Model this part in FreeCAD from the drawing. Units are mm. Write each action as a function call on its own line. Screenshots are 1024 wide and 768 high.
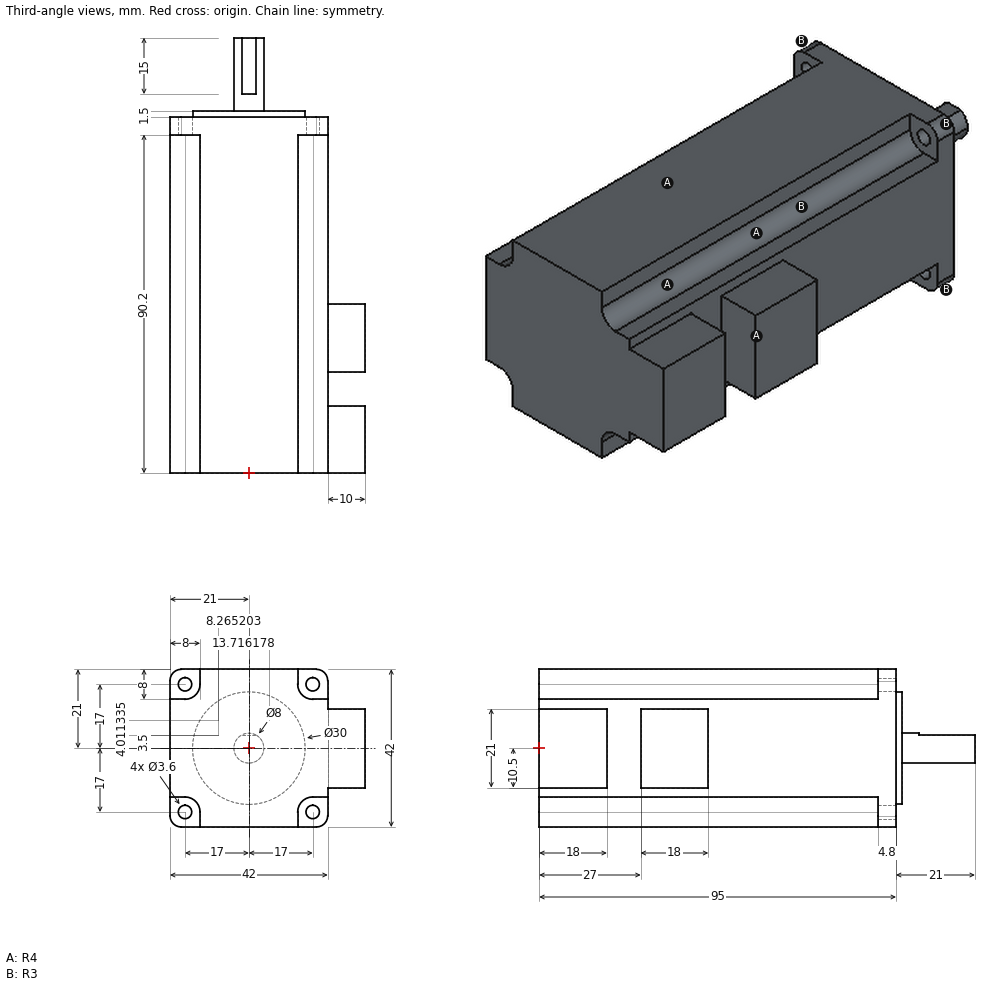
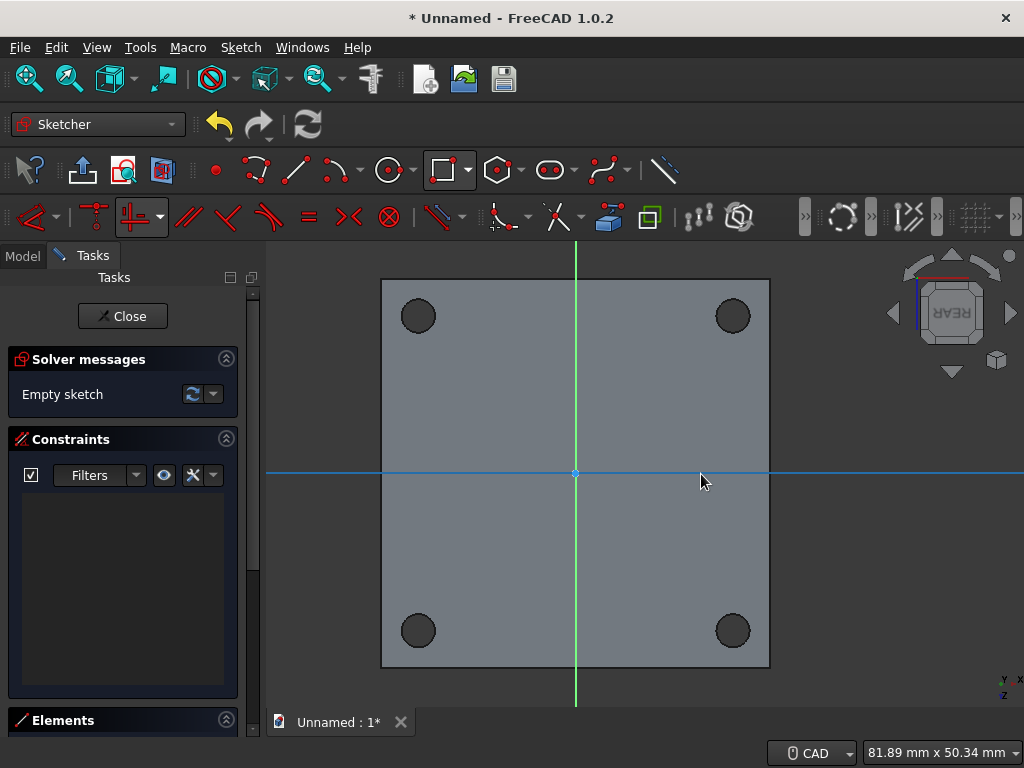
key(g)
key(c)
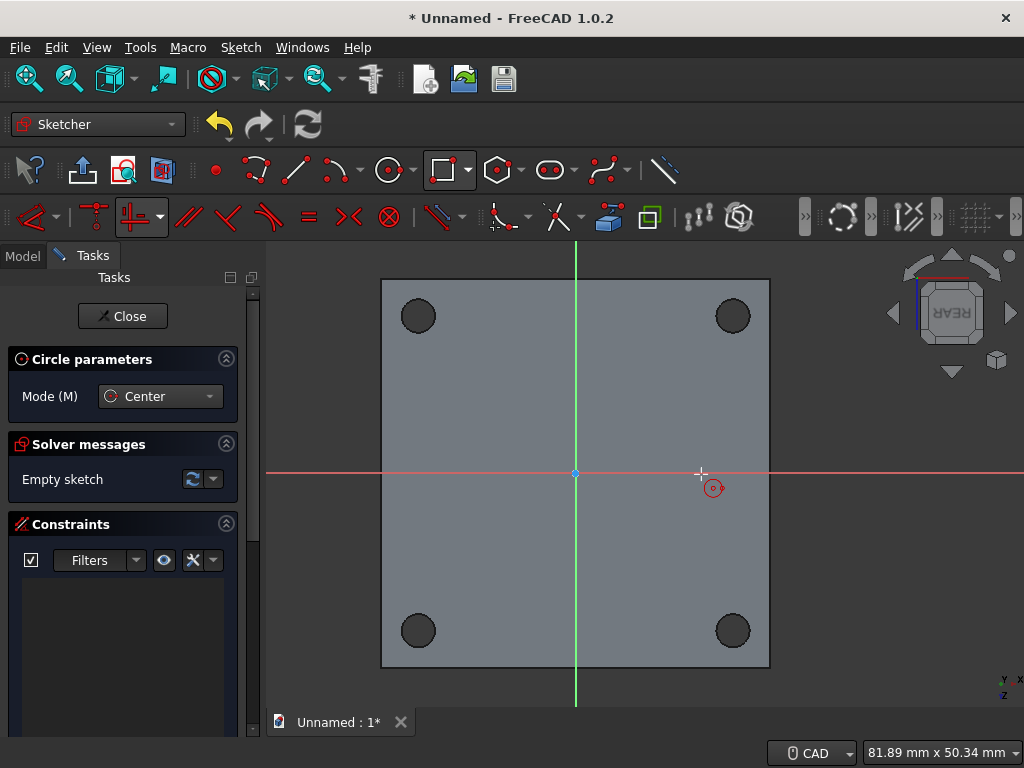
click(576, 473)
click(674, 375)
key(Escape)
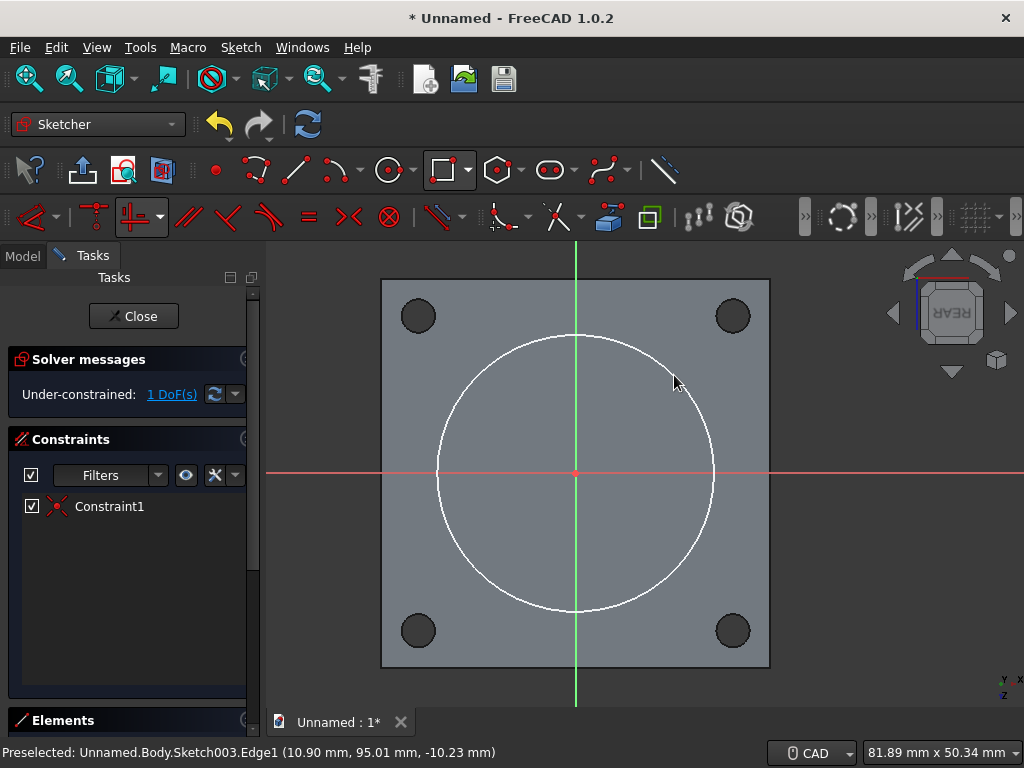
click(32, 218)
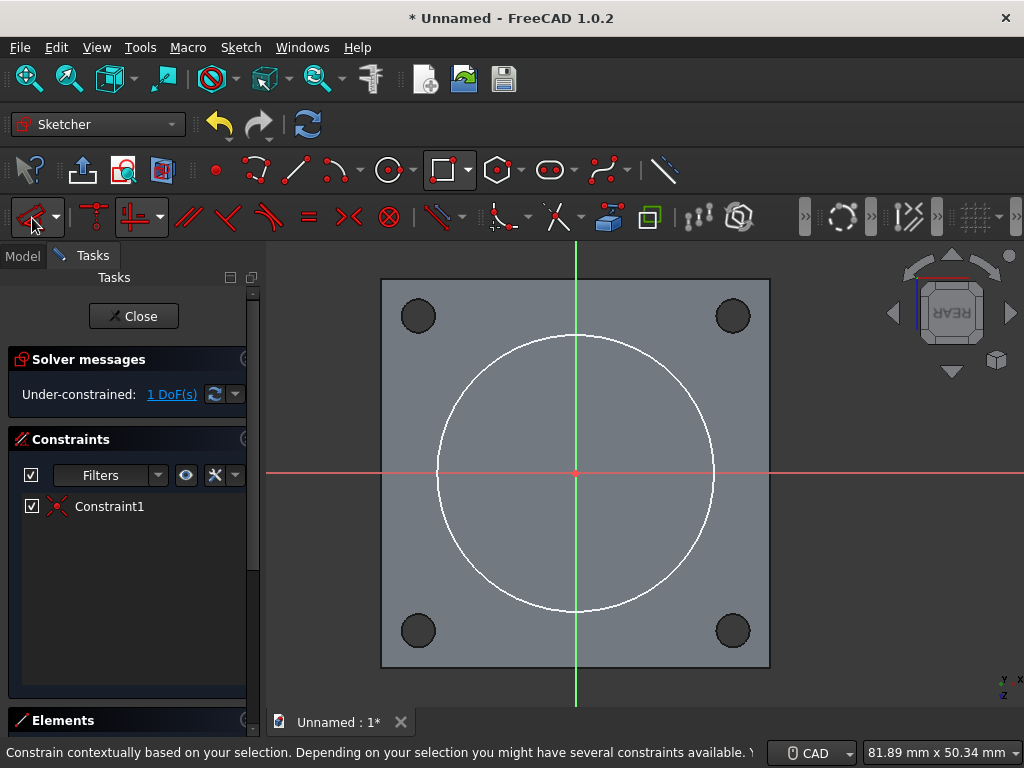
click(673, 375)
click(696, 352)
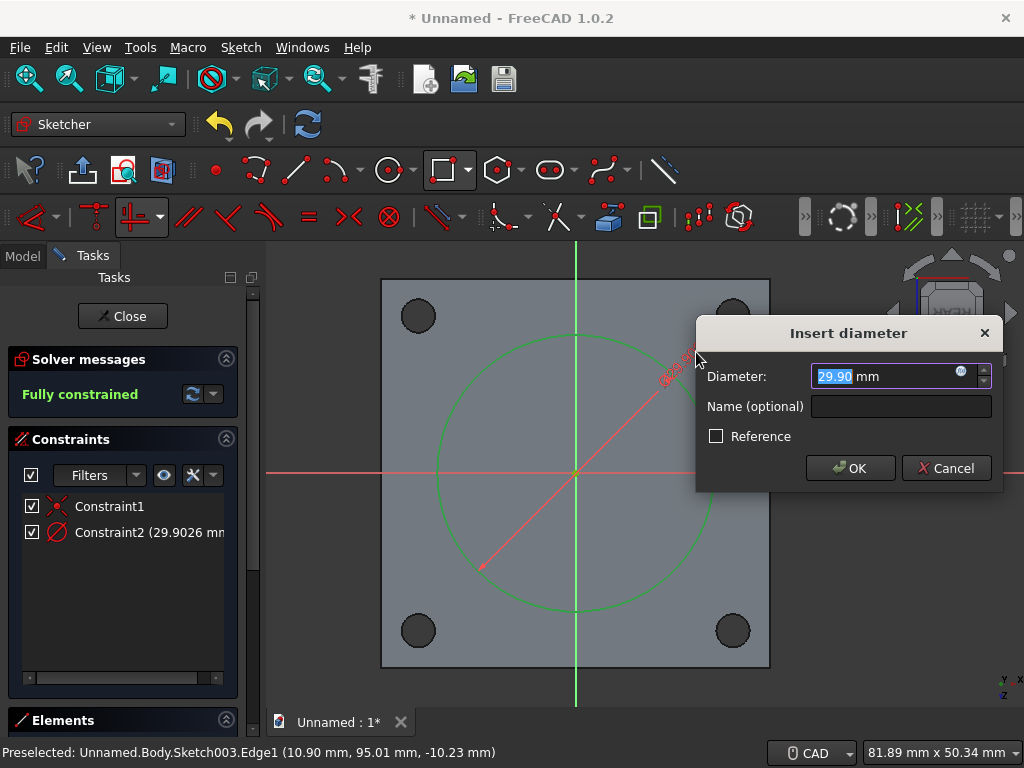
text(30)
key(Return)
key(Escape)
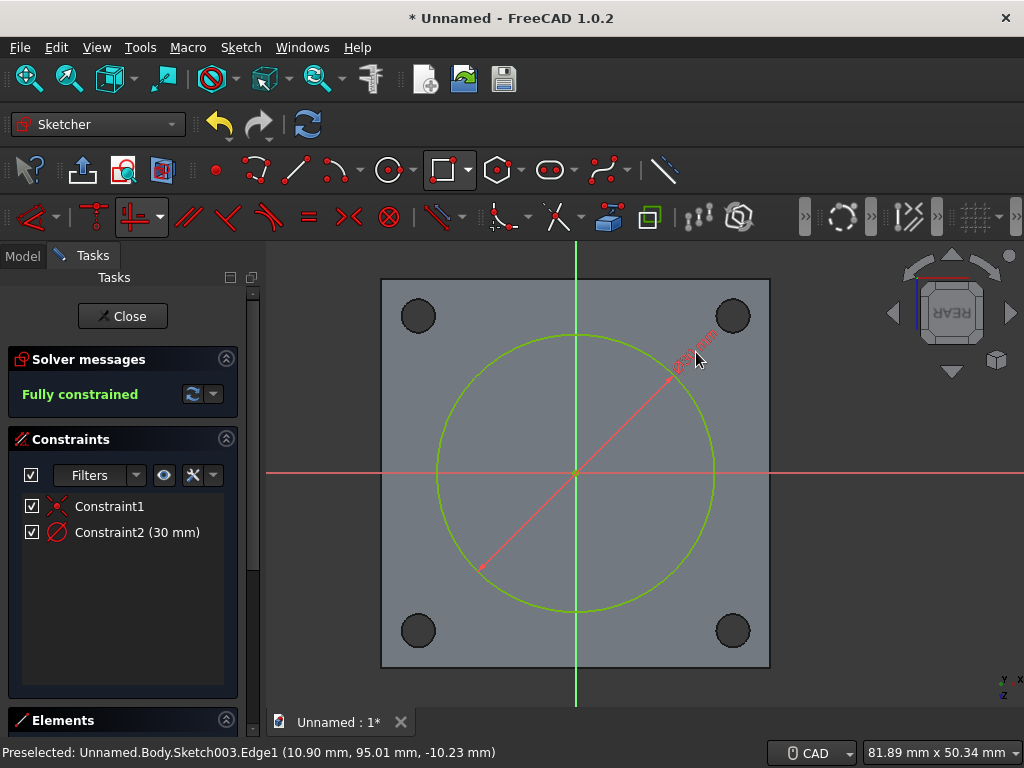
click(123, 316)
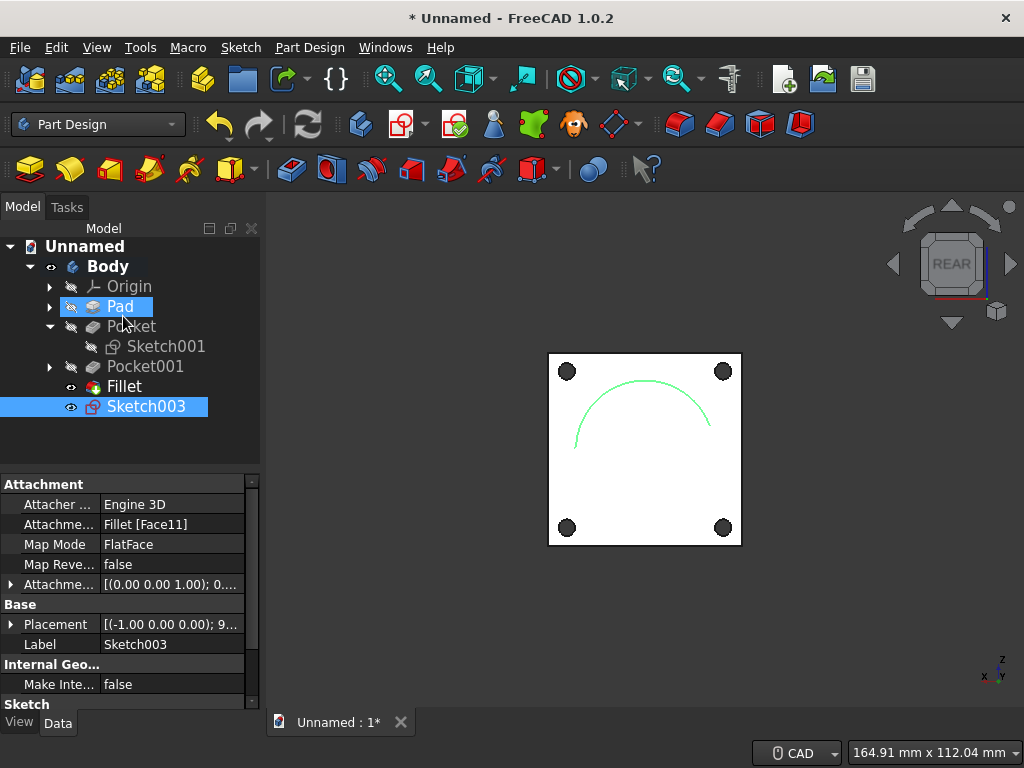
click(30, 170)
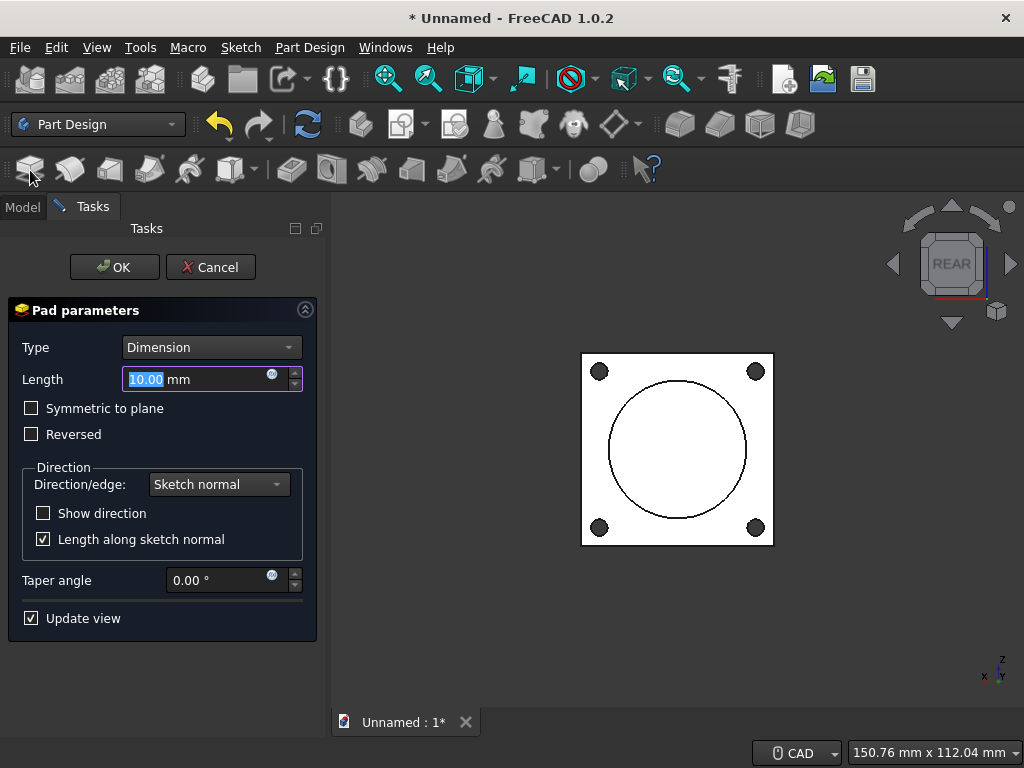
text(1.5)
key(Tab)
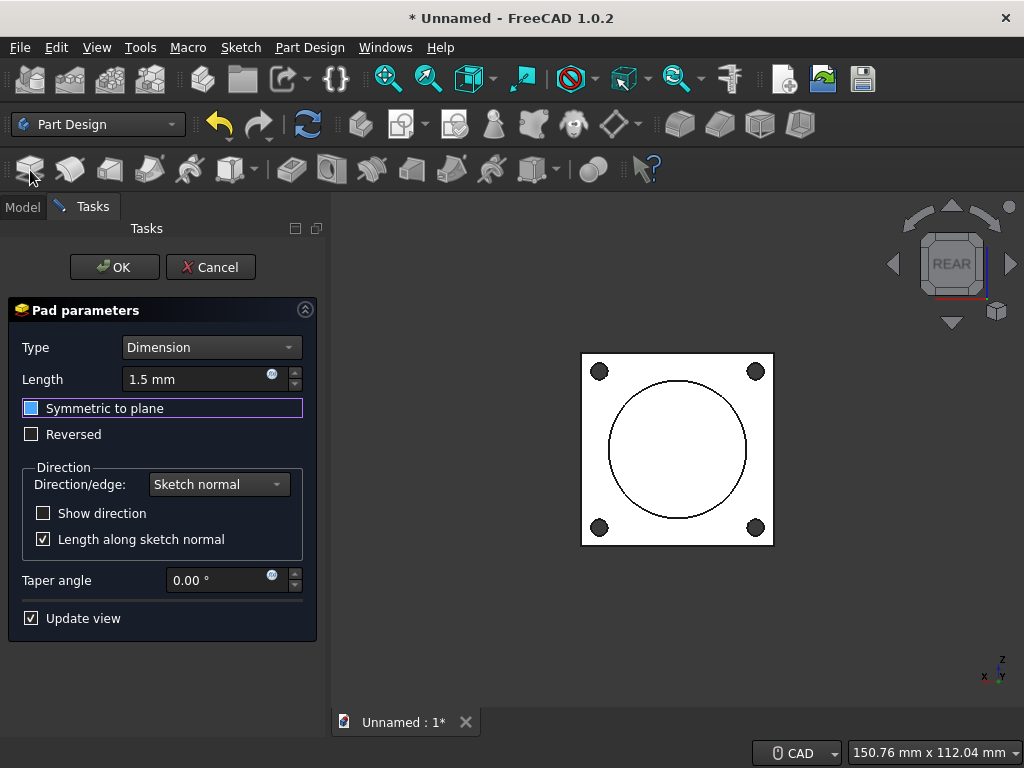
click(115, 267)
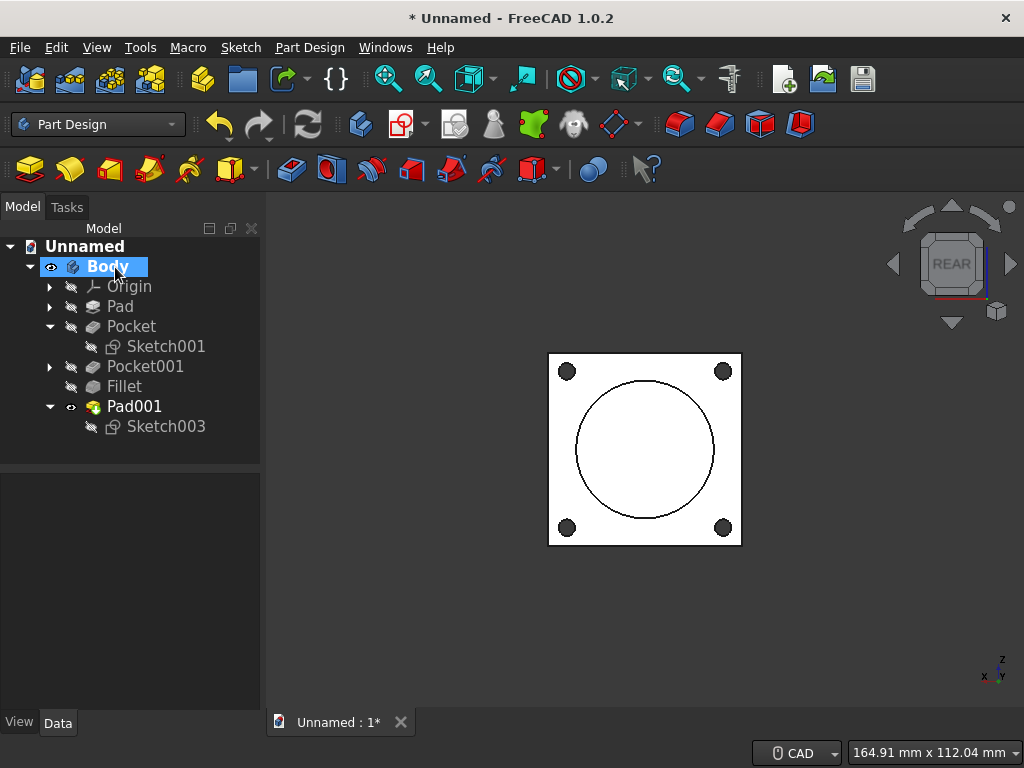
key(v)
key(f)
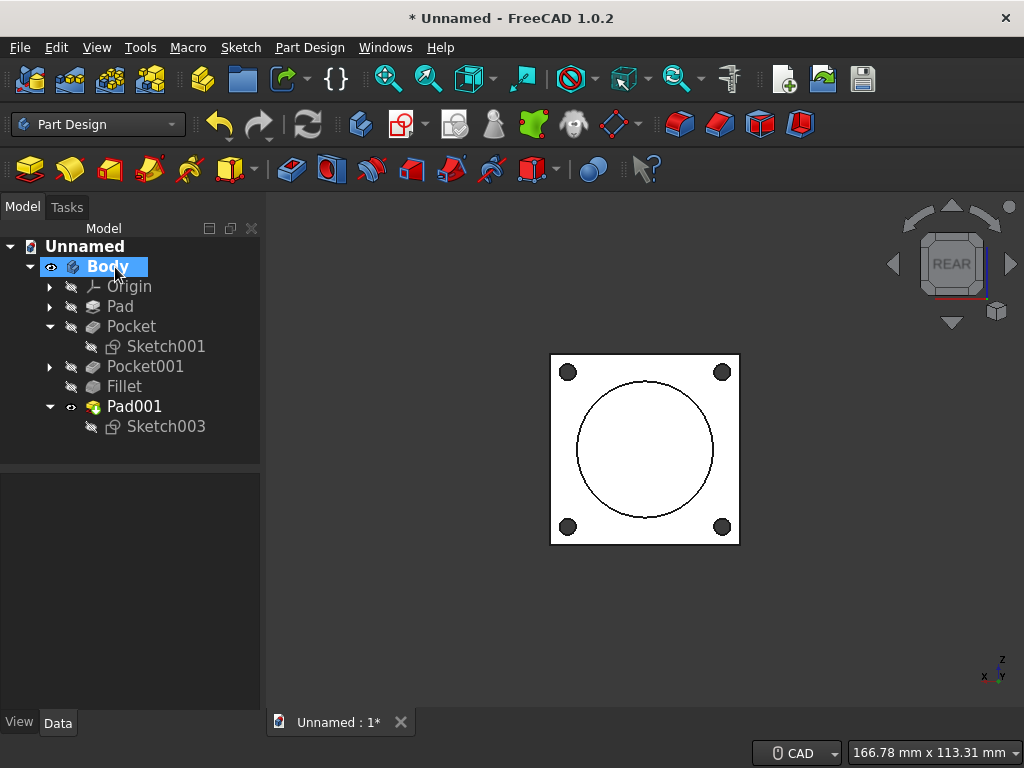
click(563, 394)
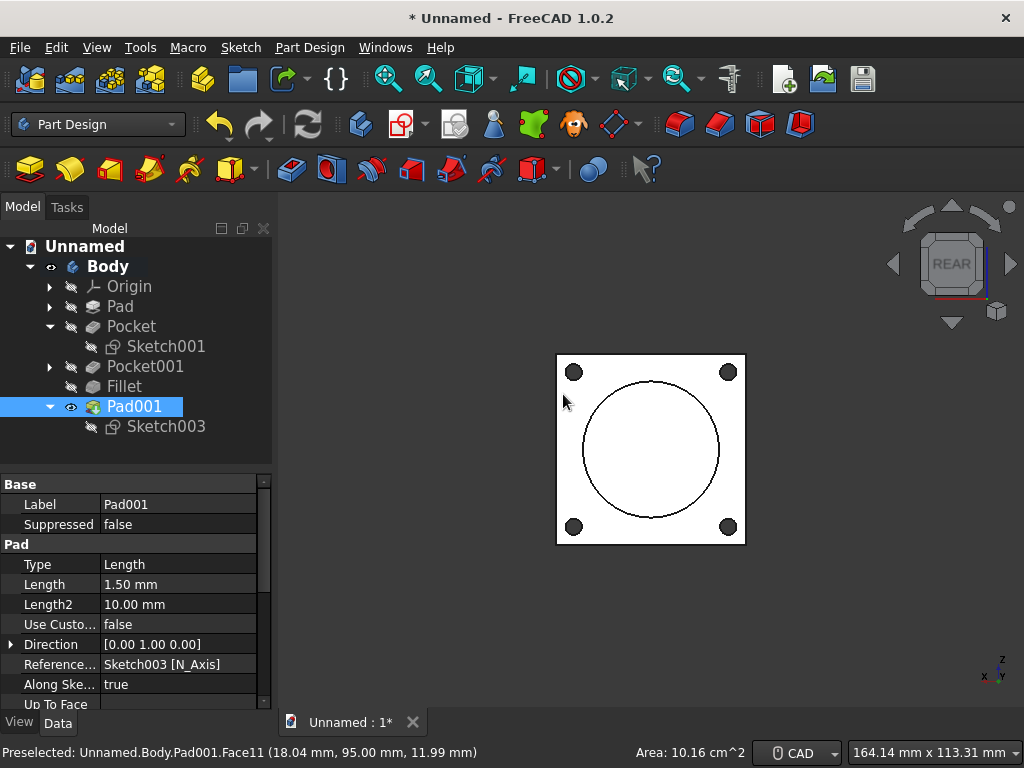
click(402, 124)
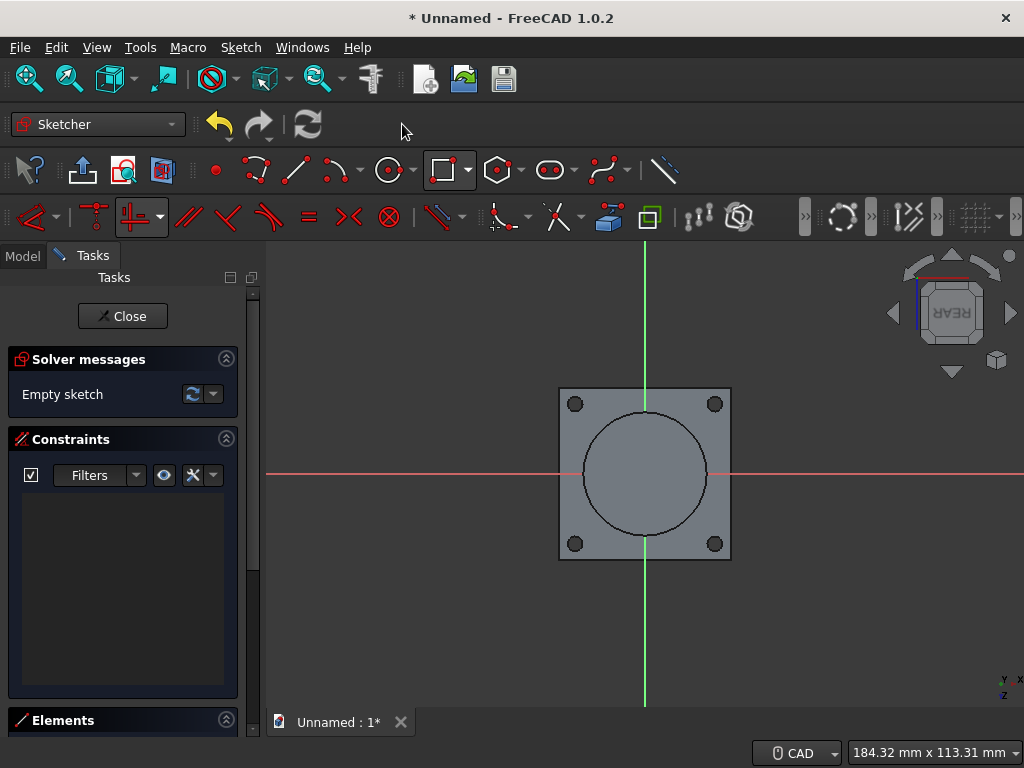
scroll(654, 474, up, 11)